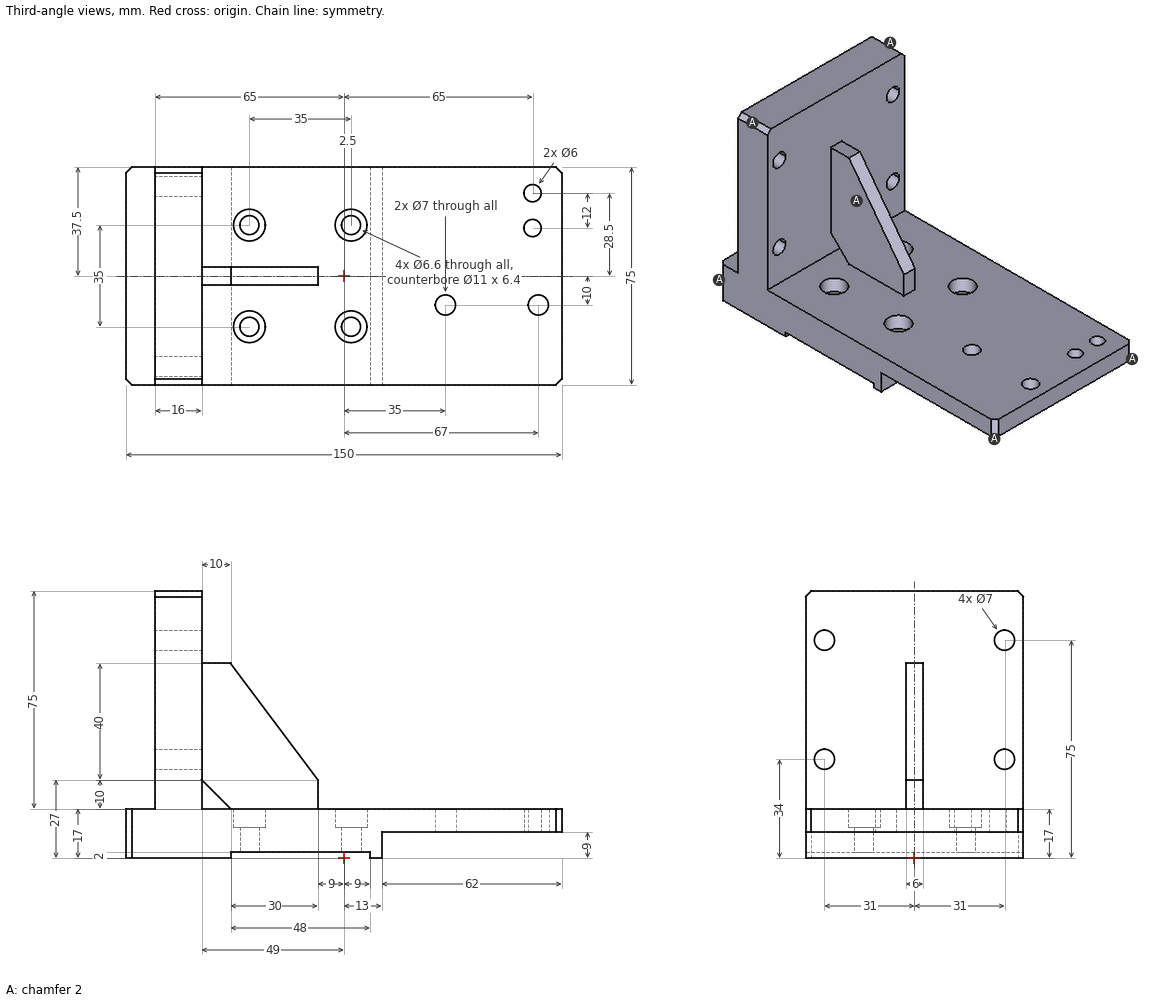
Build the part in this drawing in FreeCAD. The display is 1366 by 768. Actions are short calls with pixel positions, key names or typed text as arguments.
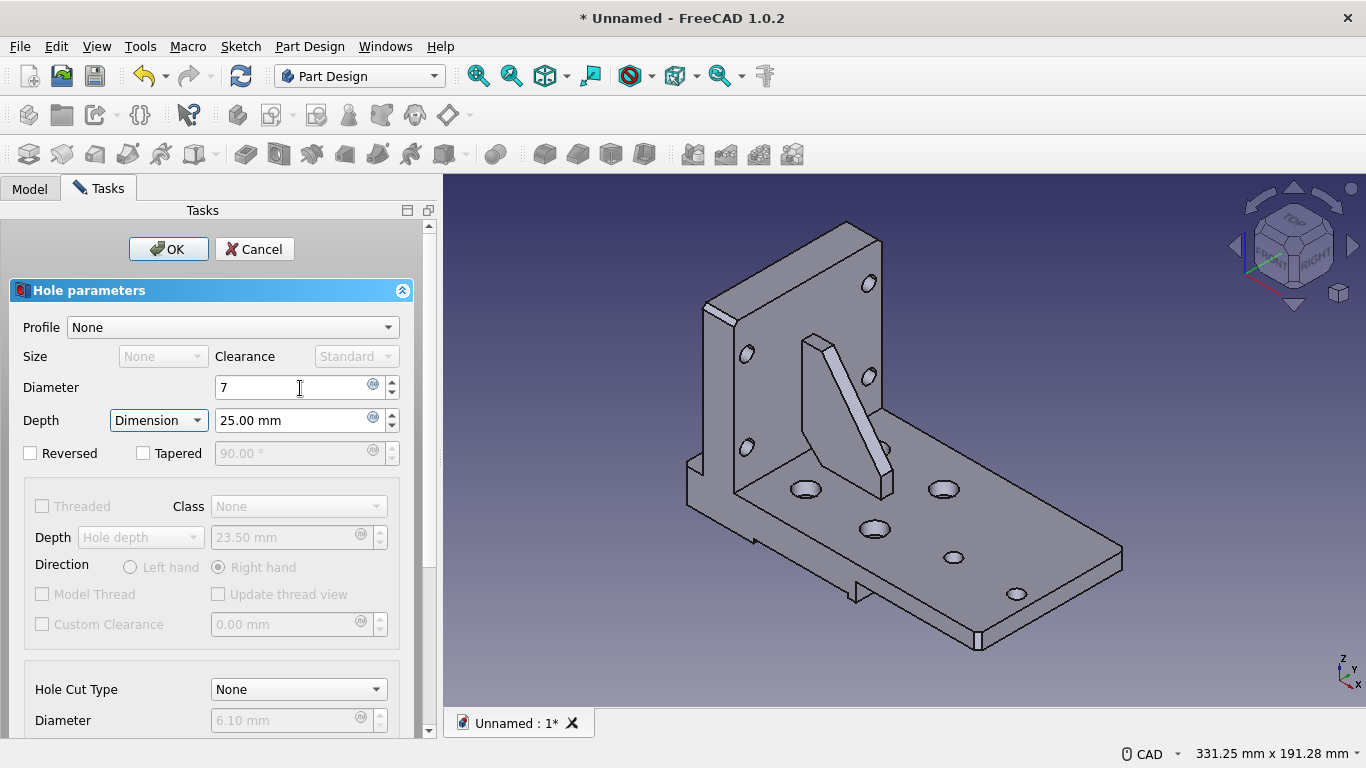
click(160, 420)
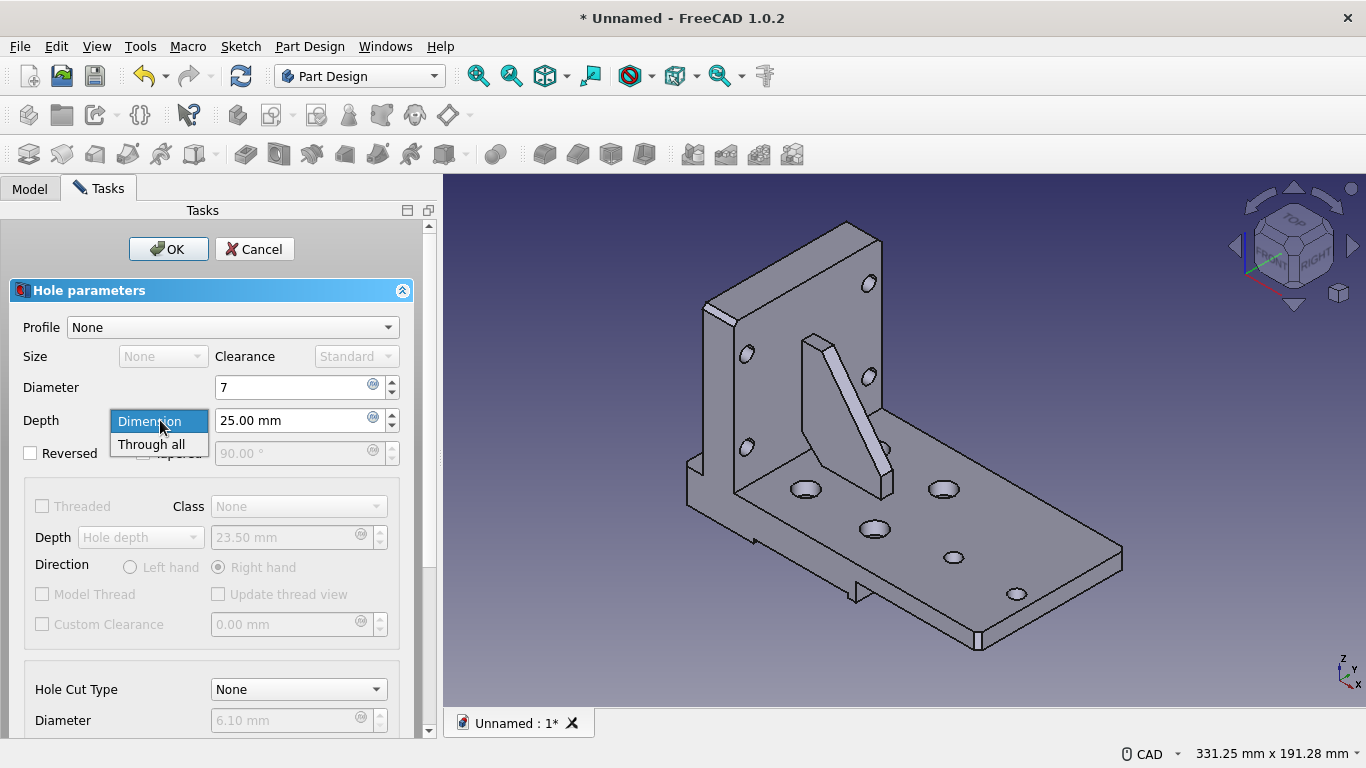
click(158, 444)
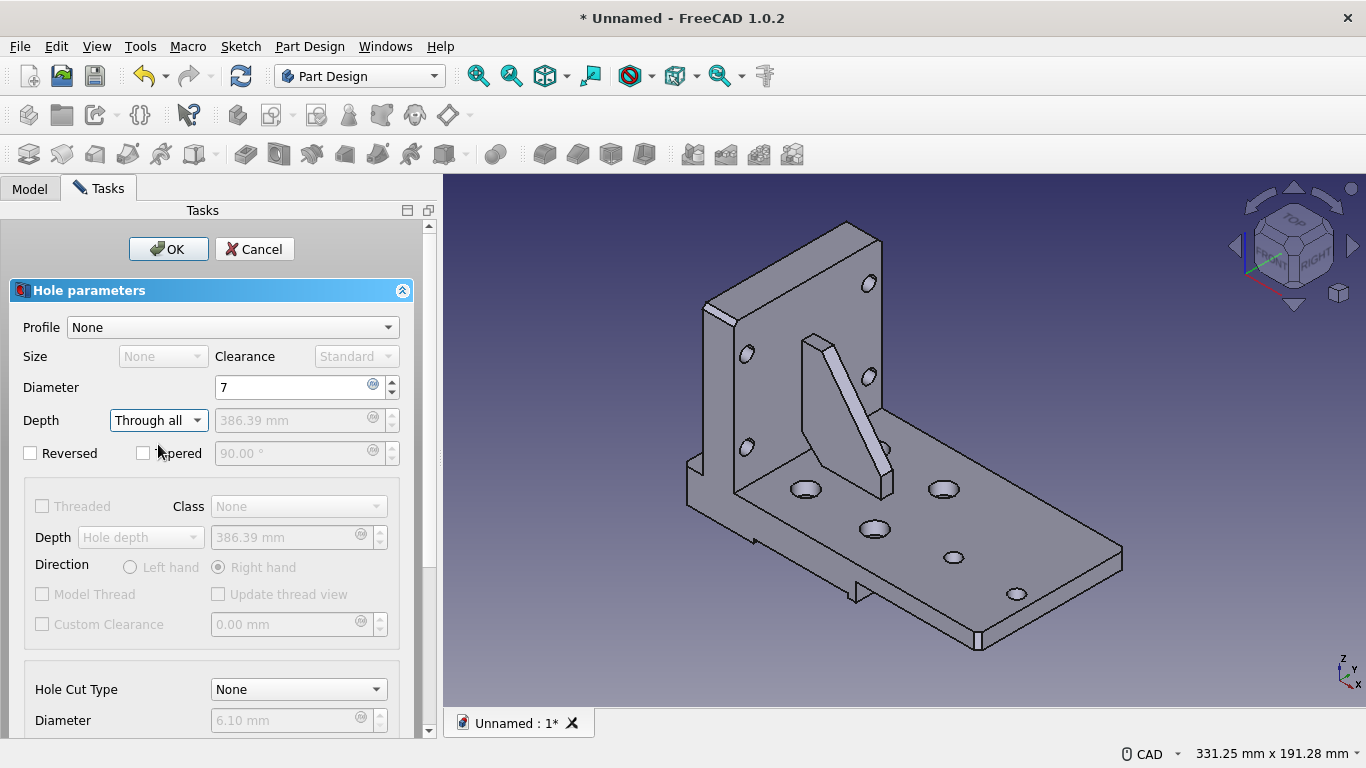
click(169, 249)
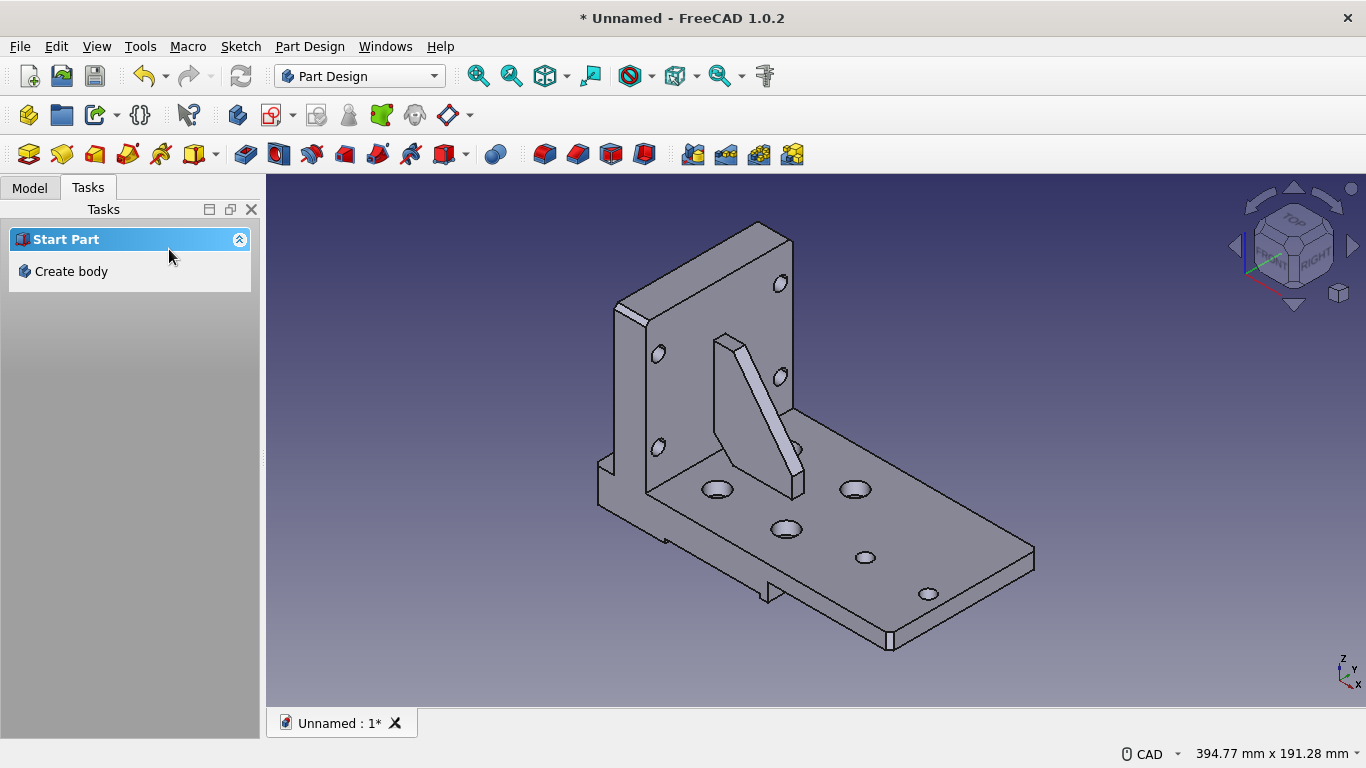
click(933, 548)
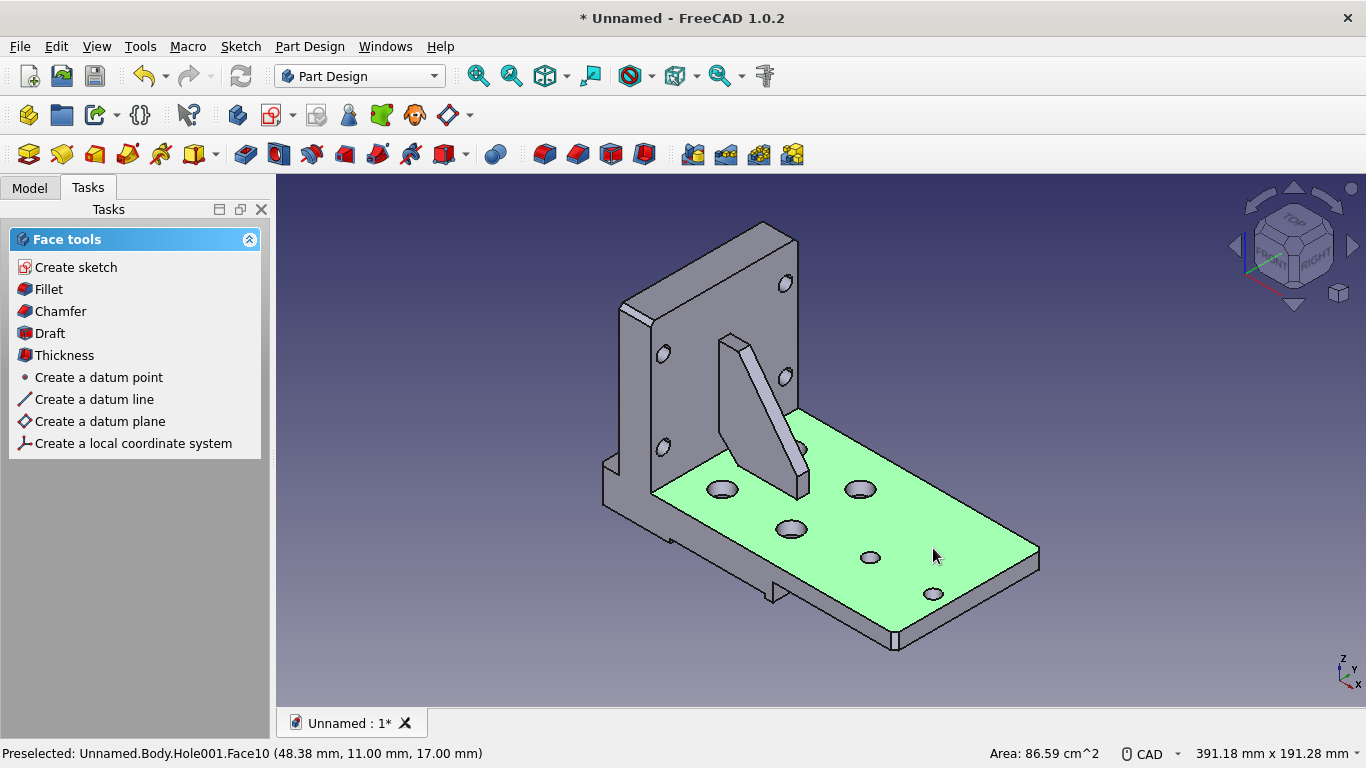
click(270, 116)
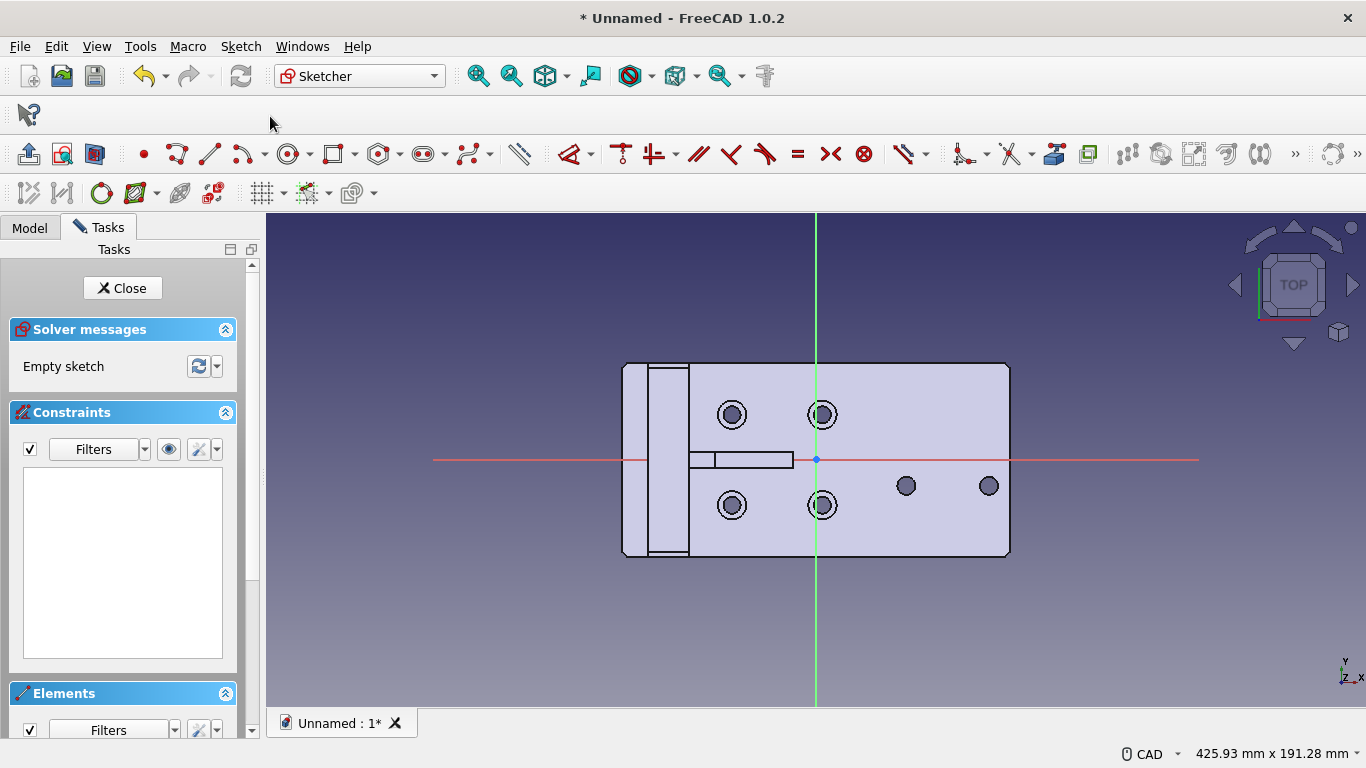
scroll(1031, 390, up, 9)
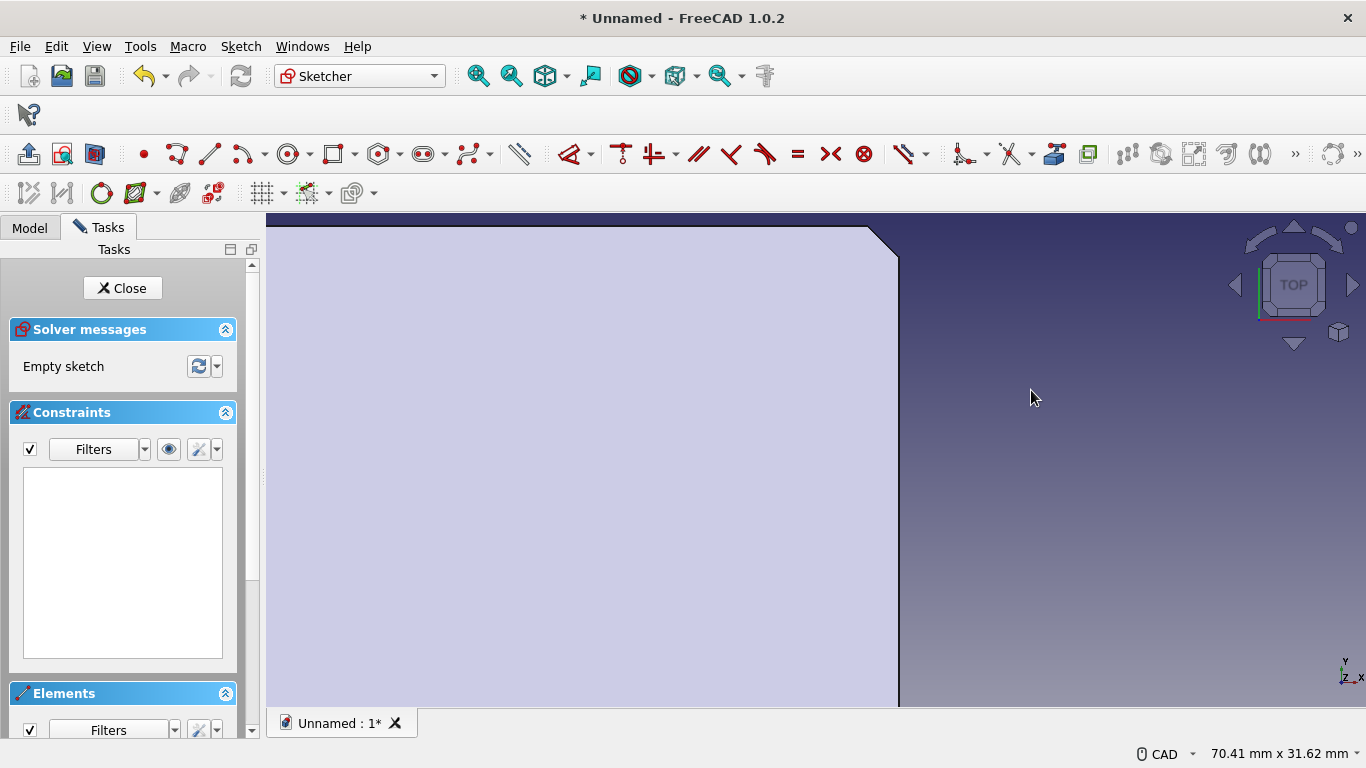
click(288, 154)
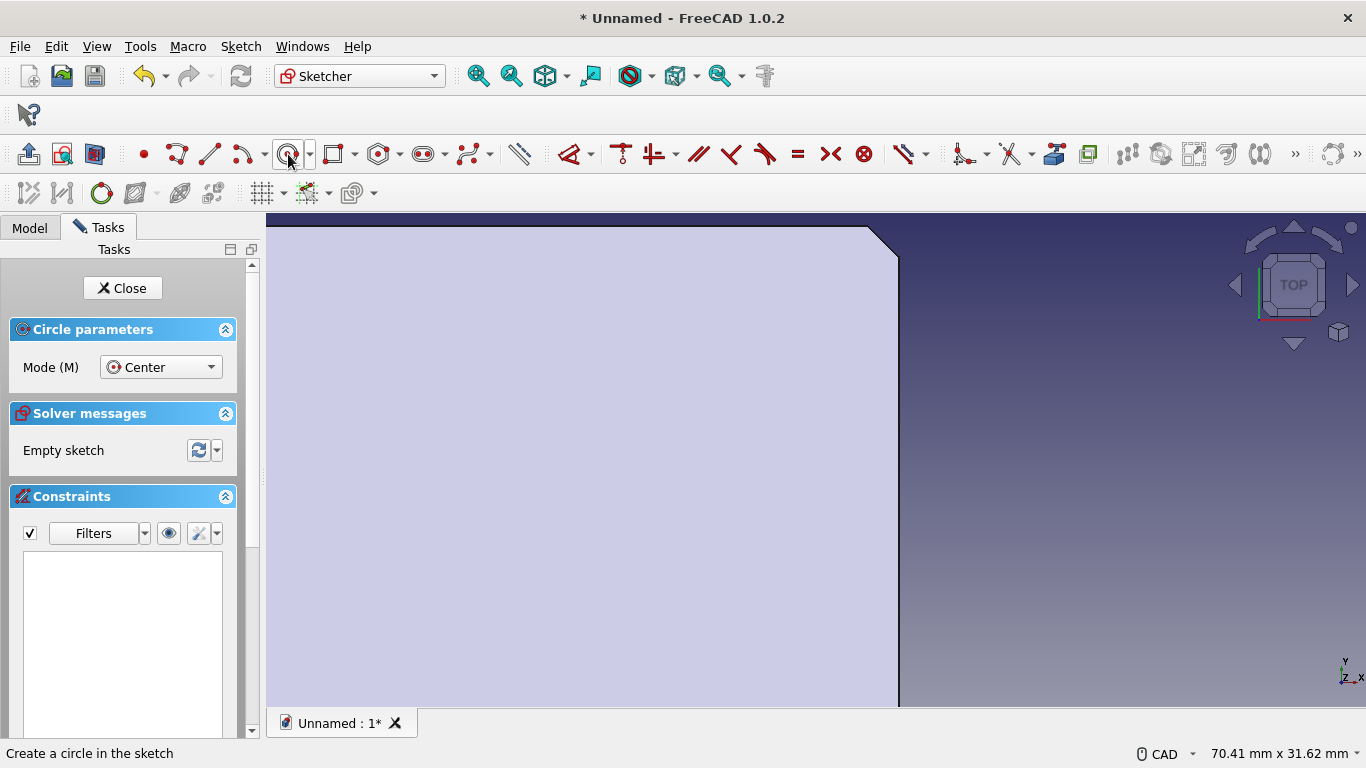
click(742, 366)
move(775, 333)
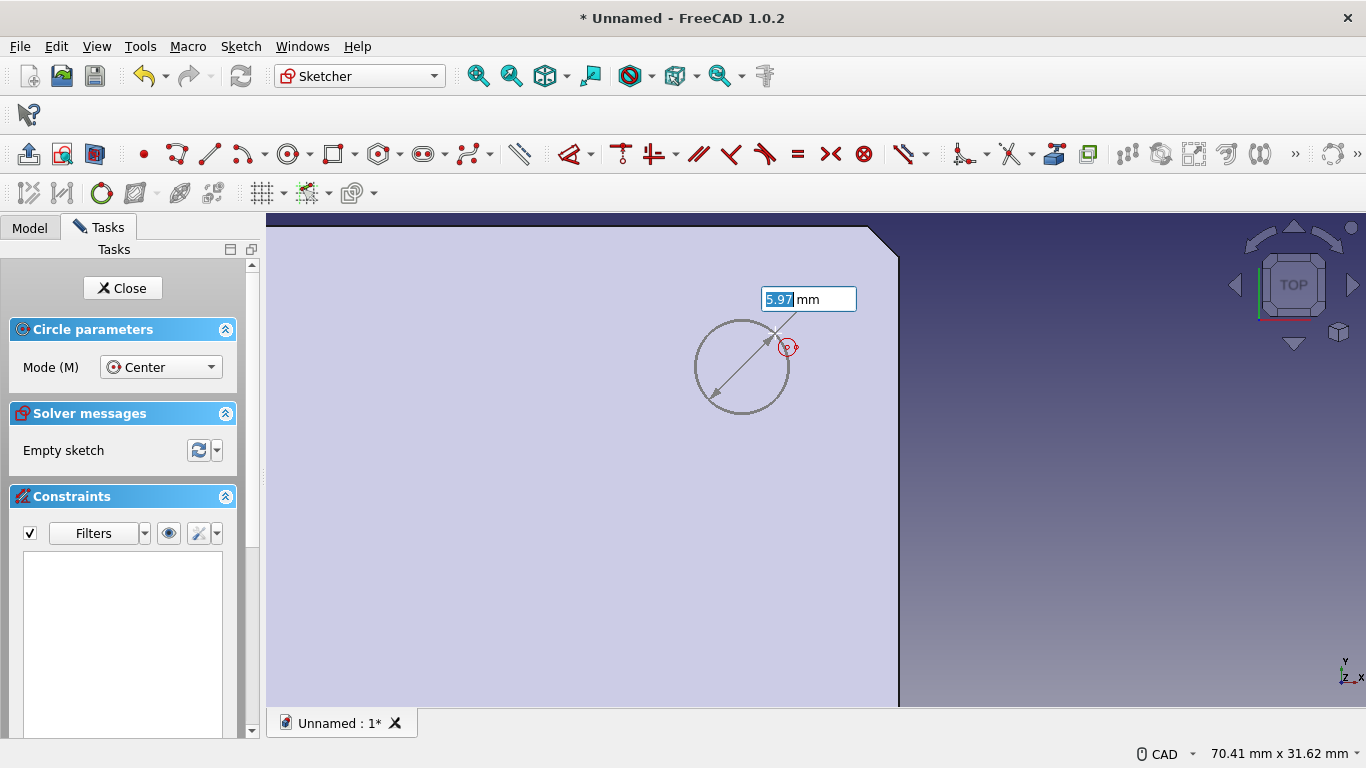
text(6)
key(Return)